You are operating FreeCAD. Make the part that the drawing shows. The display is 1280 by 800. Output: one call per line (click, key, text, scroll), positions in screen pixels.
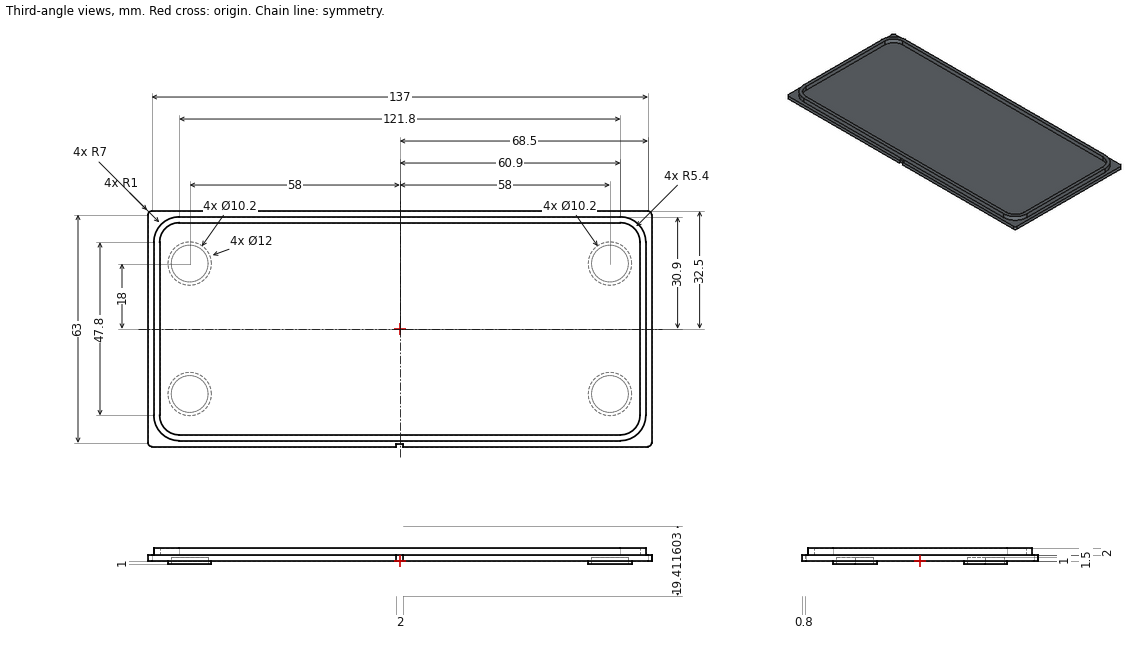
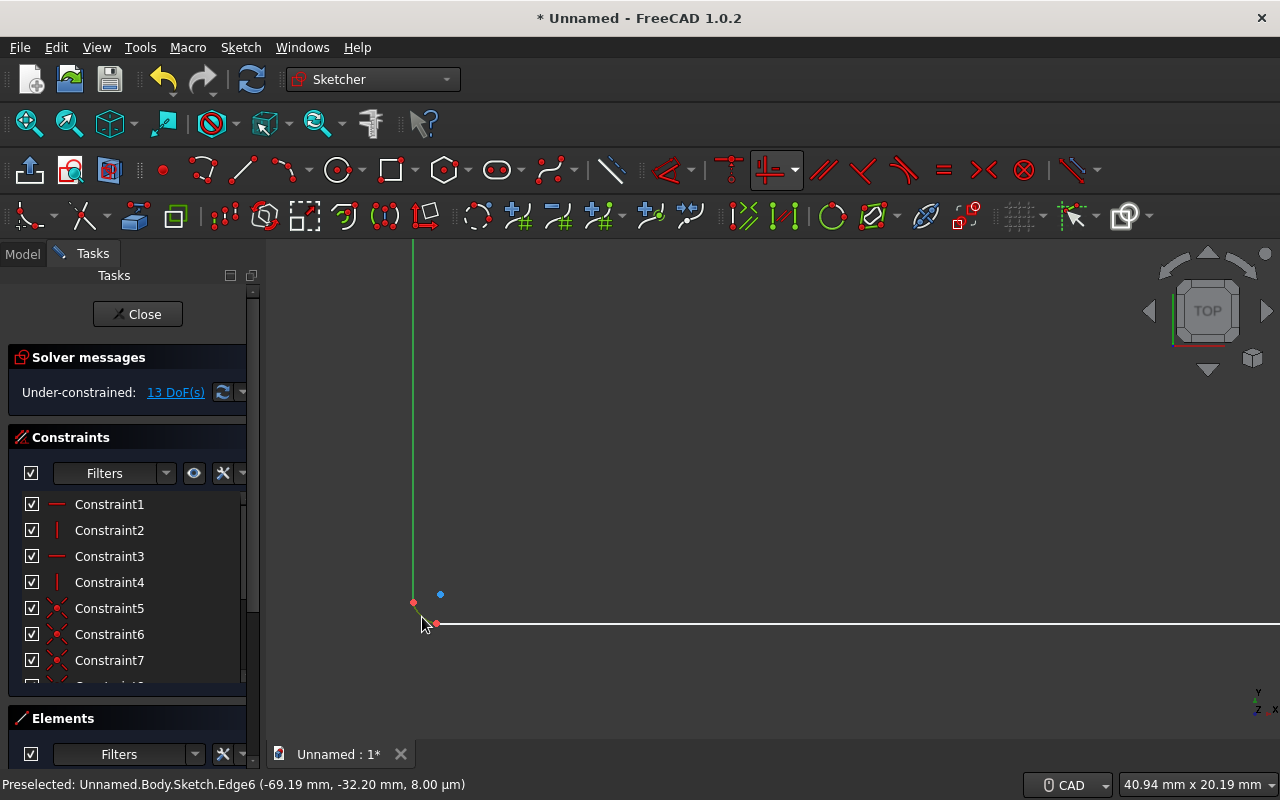
click(904, 170)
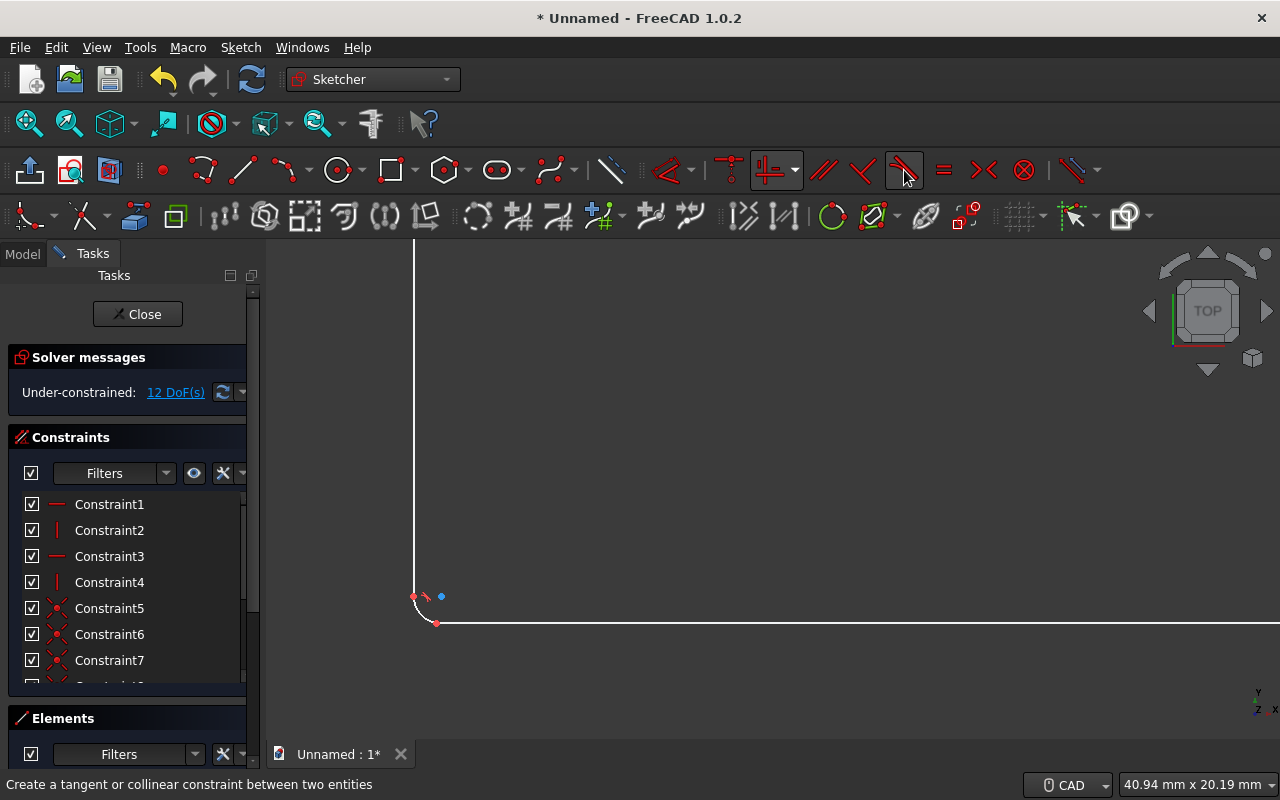
scroll(422, 622, down, 9)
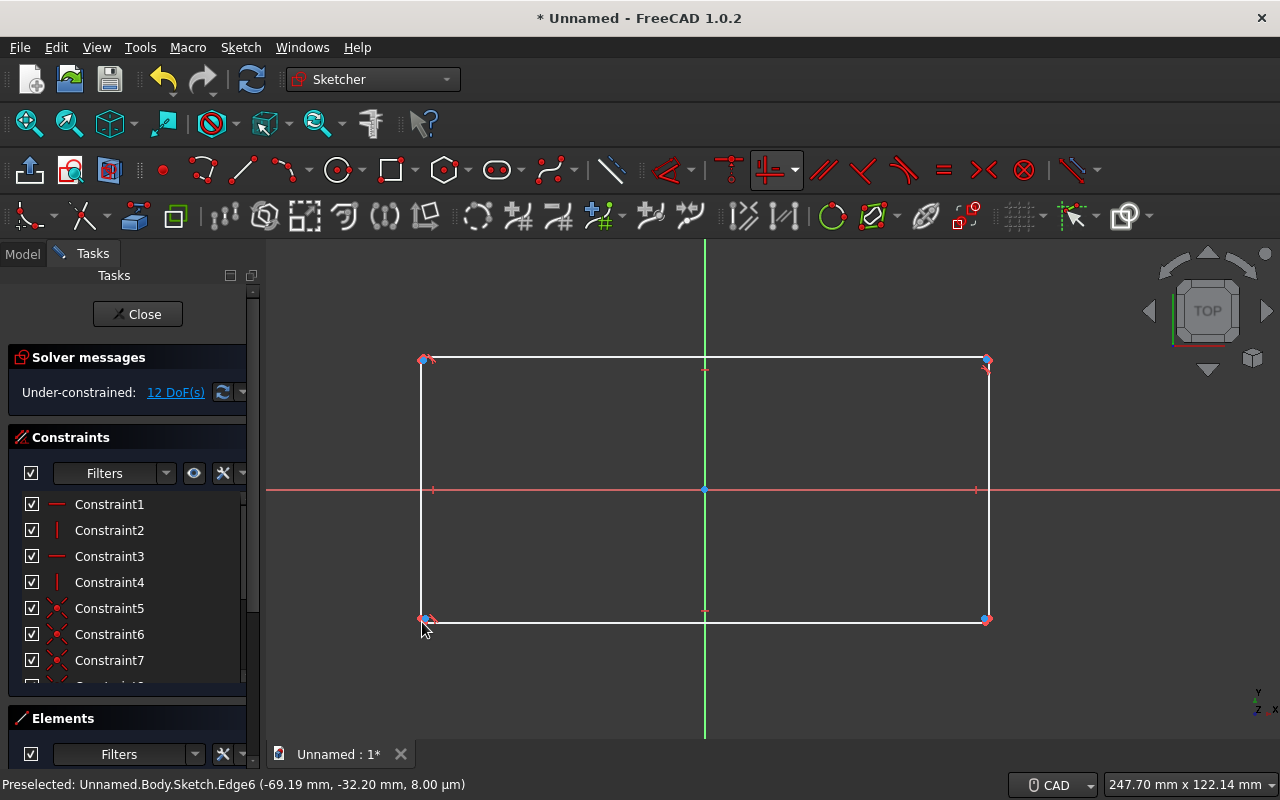
click(593, 623)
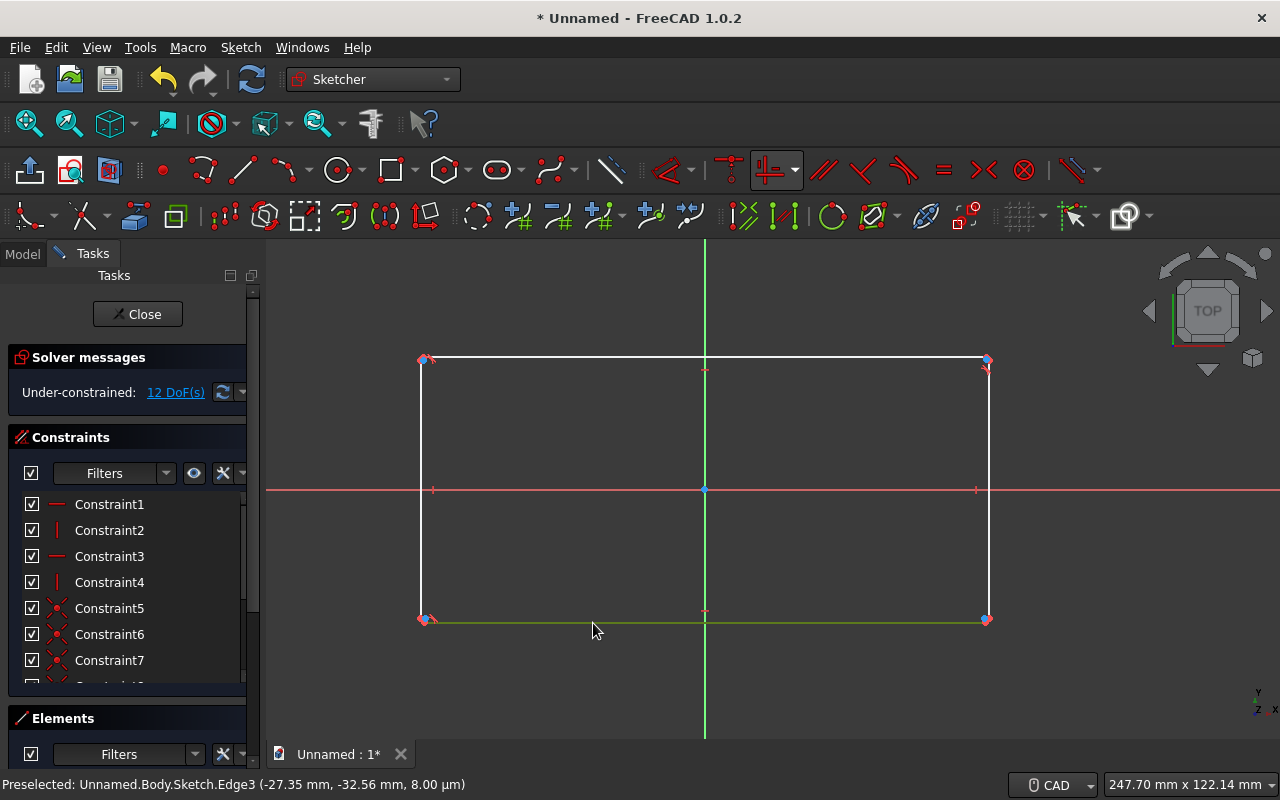
scroll(422, 621, up, 8)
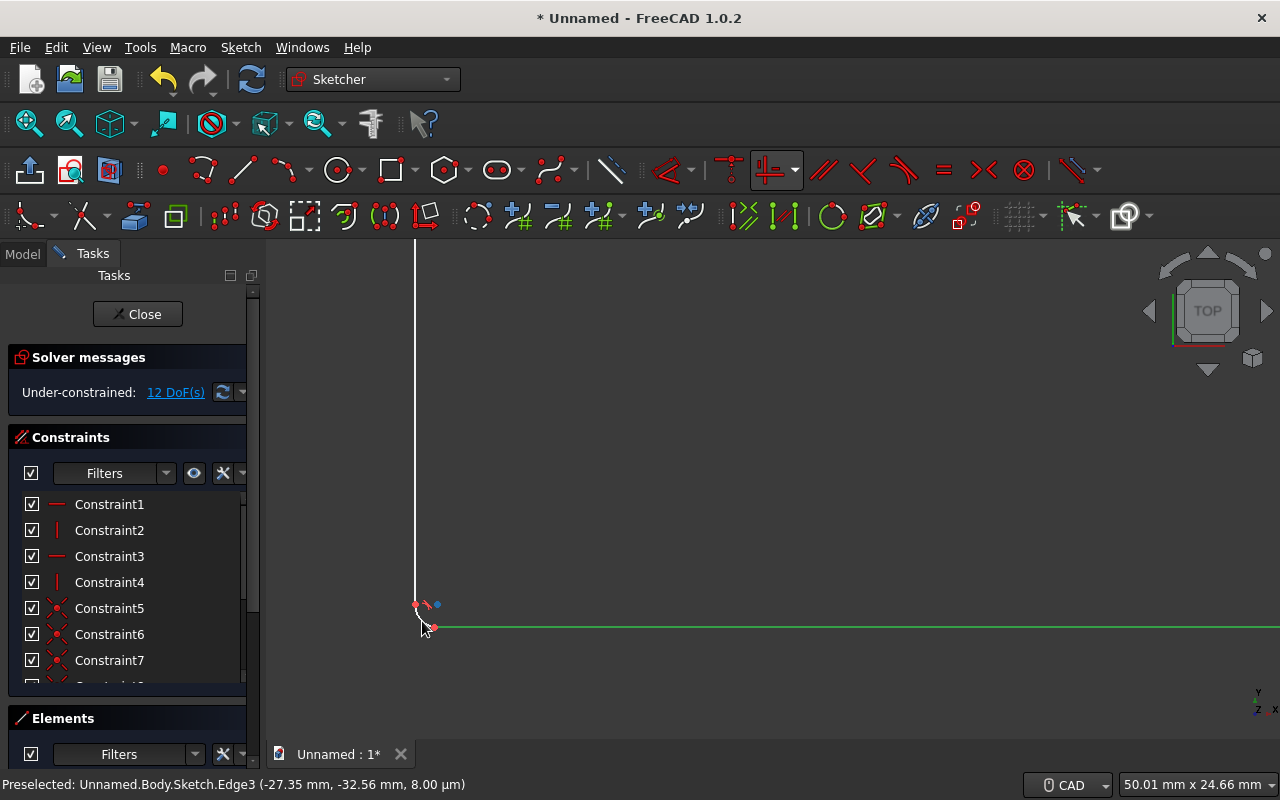
click(421, 619)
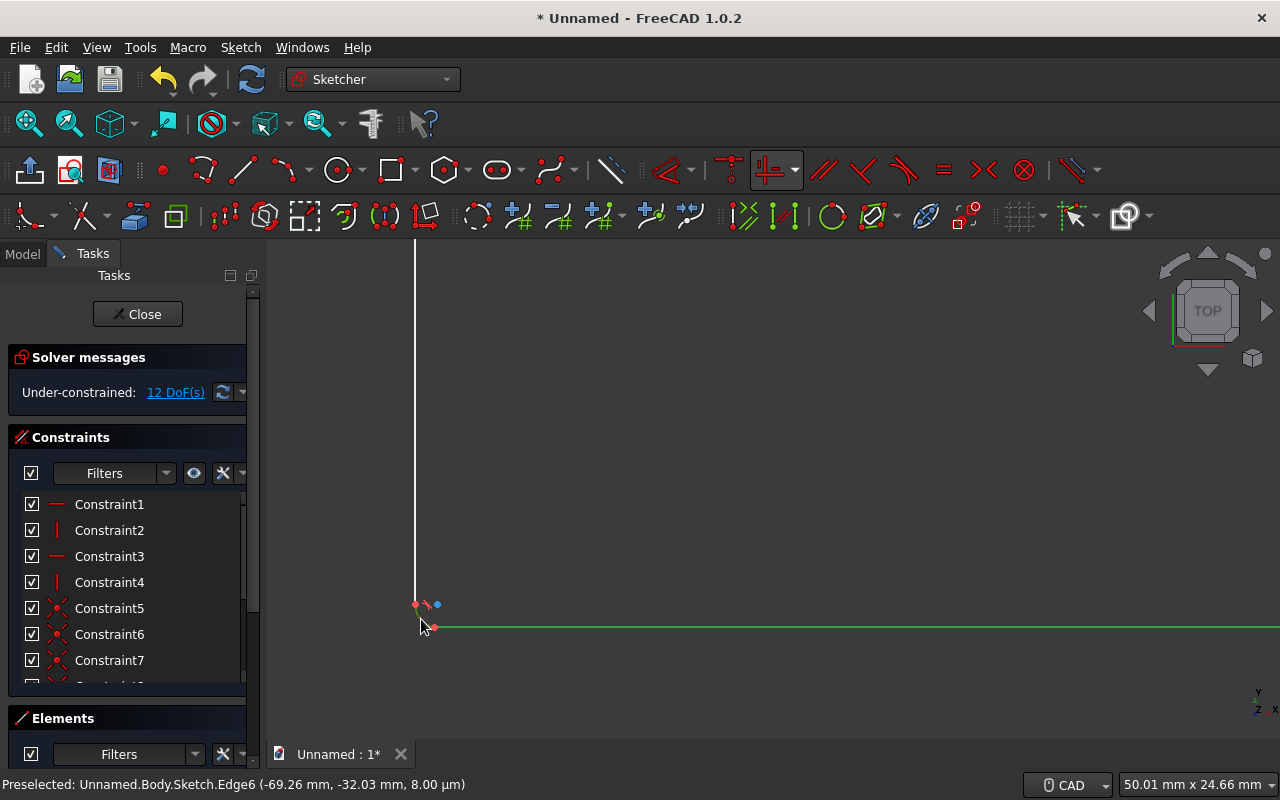
click(904, 170)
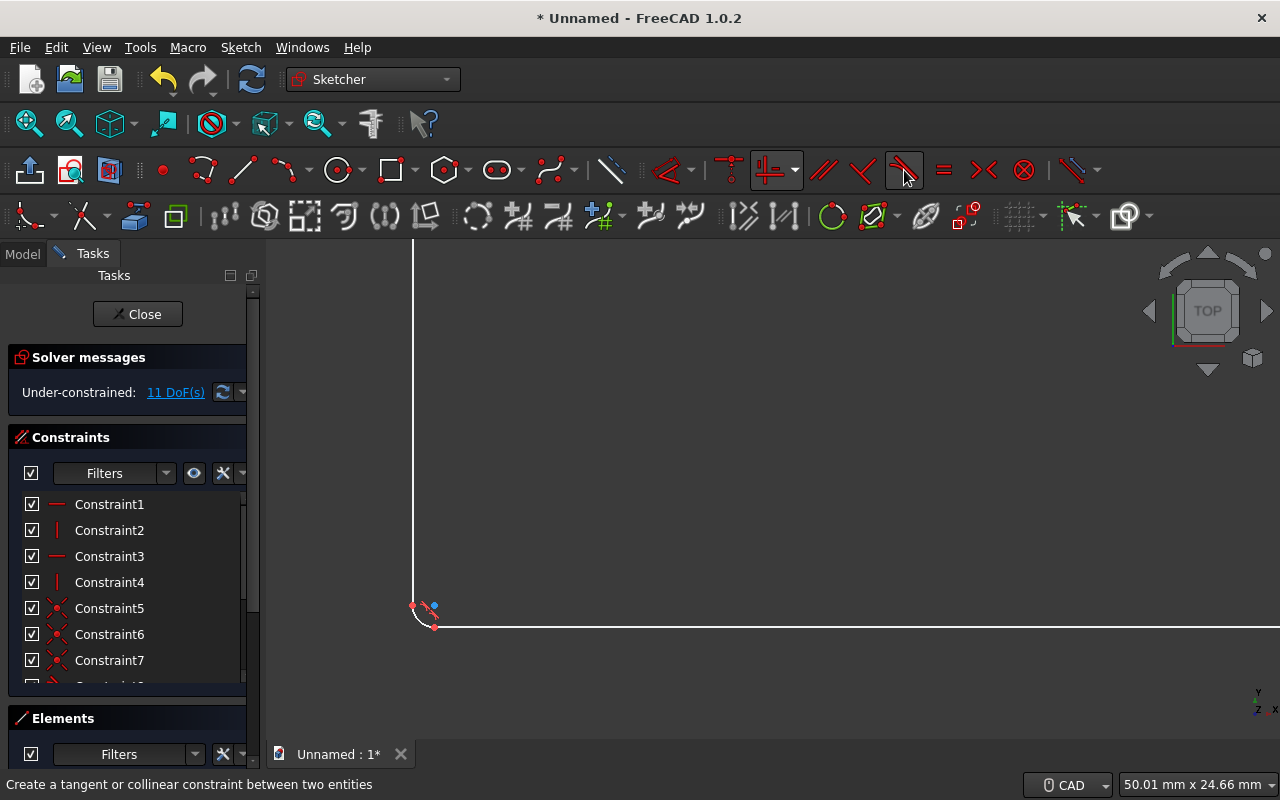
scroll(422, 621, down, 8)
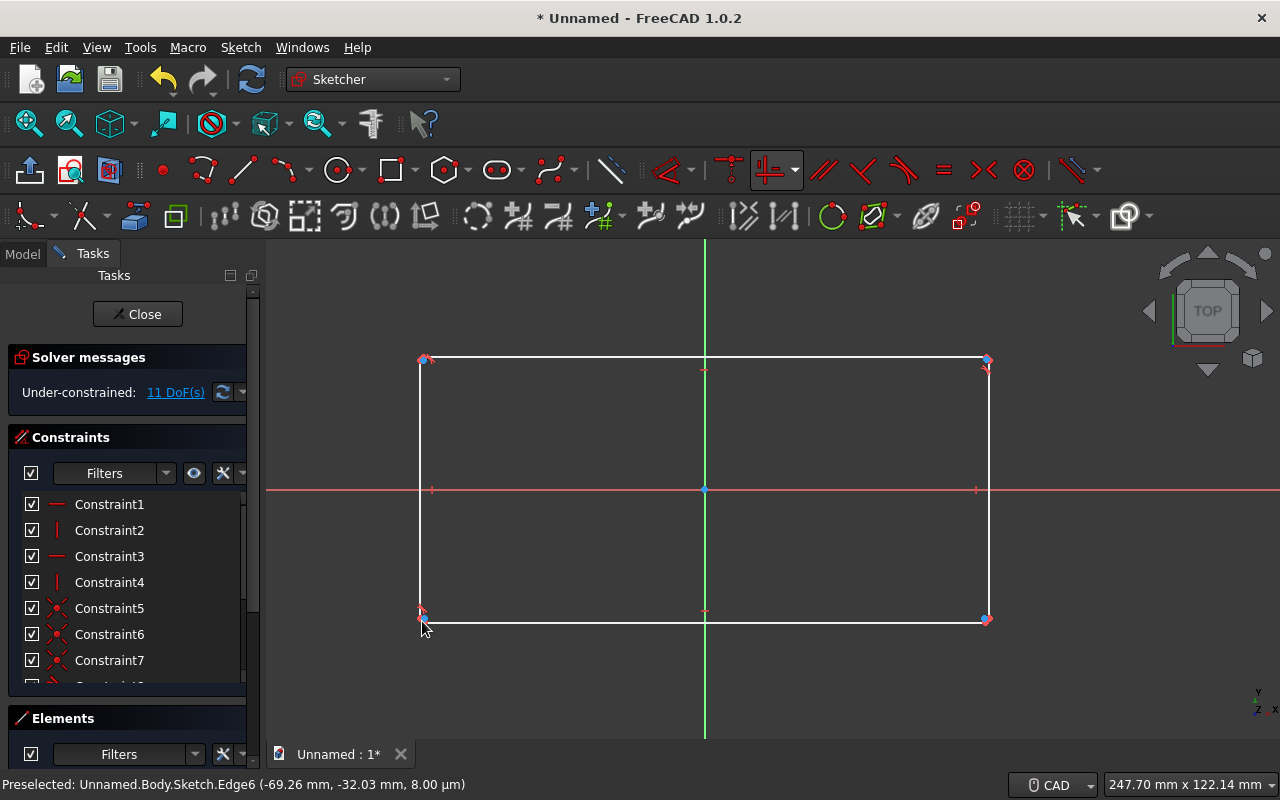
click(537, 623)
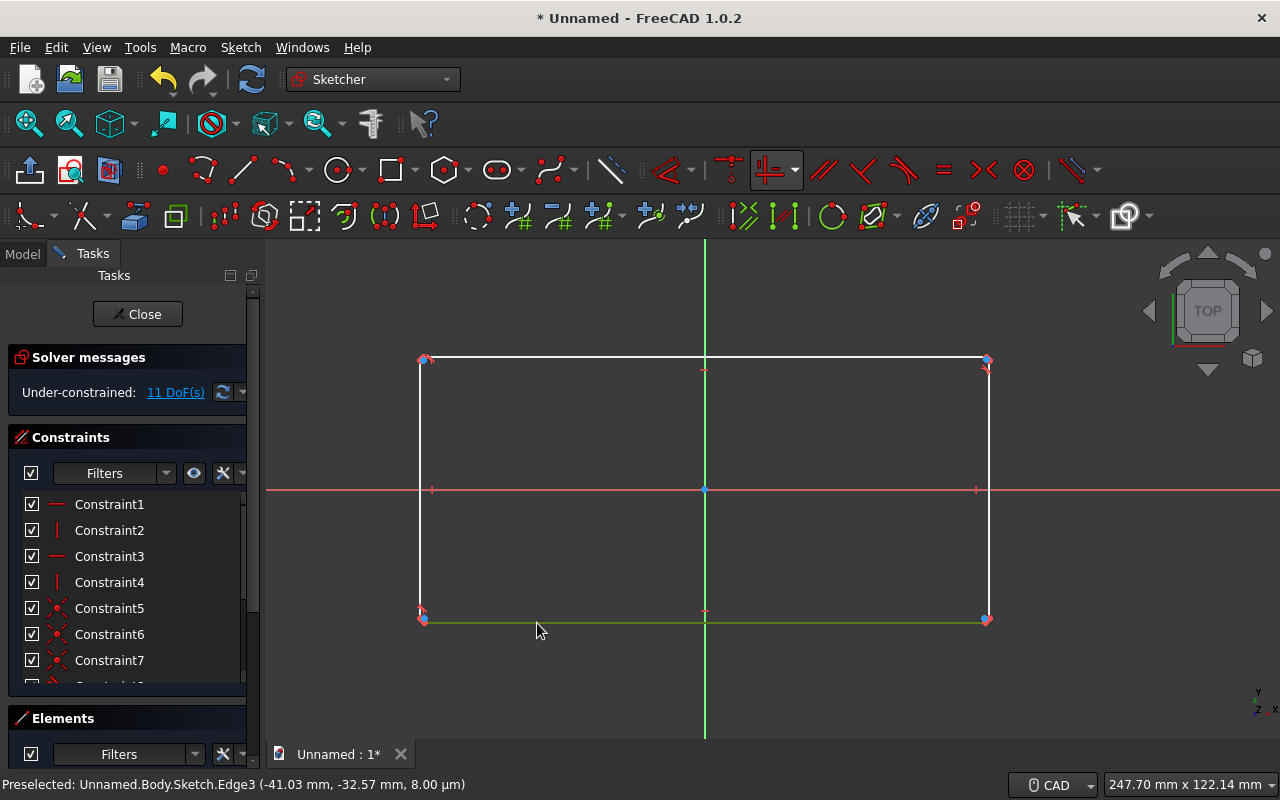
scroll(988, 621, up, 8)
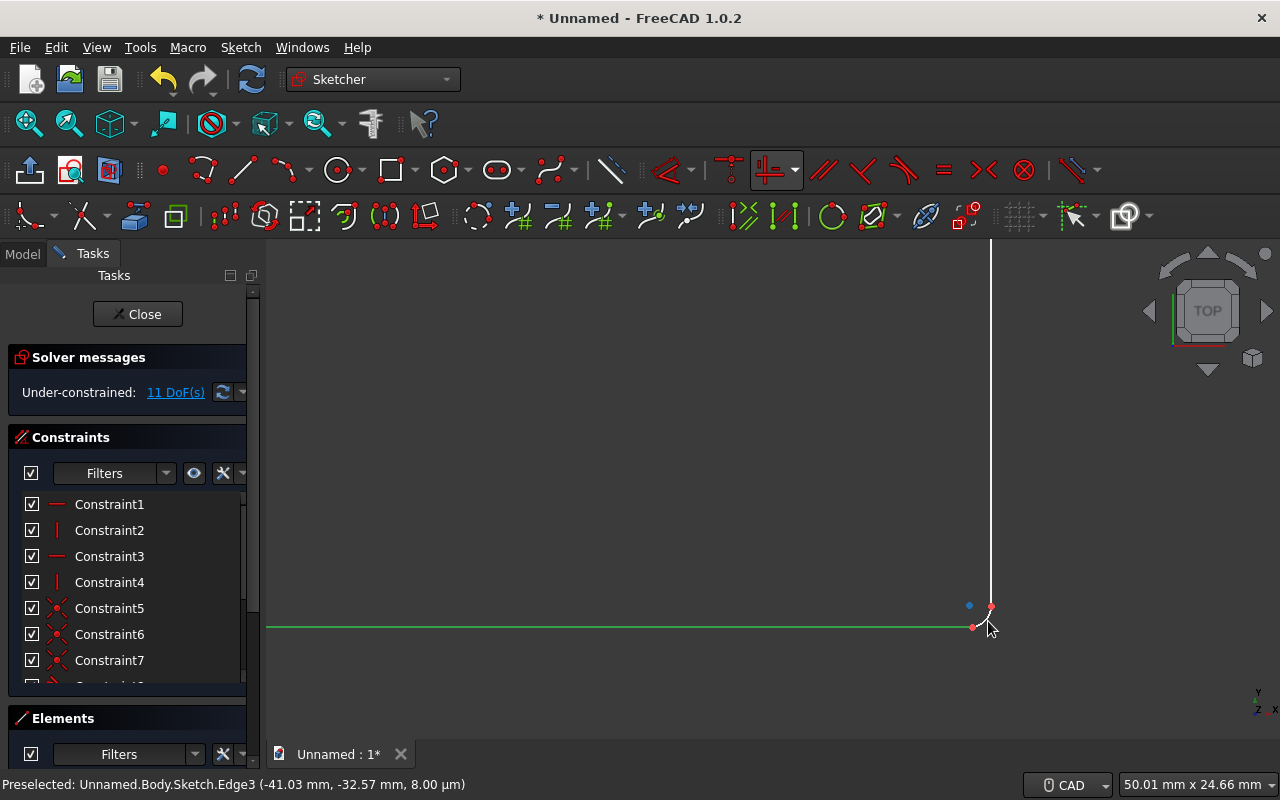
click(986, 620)